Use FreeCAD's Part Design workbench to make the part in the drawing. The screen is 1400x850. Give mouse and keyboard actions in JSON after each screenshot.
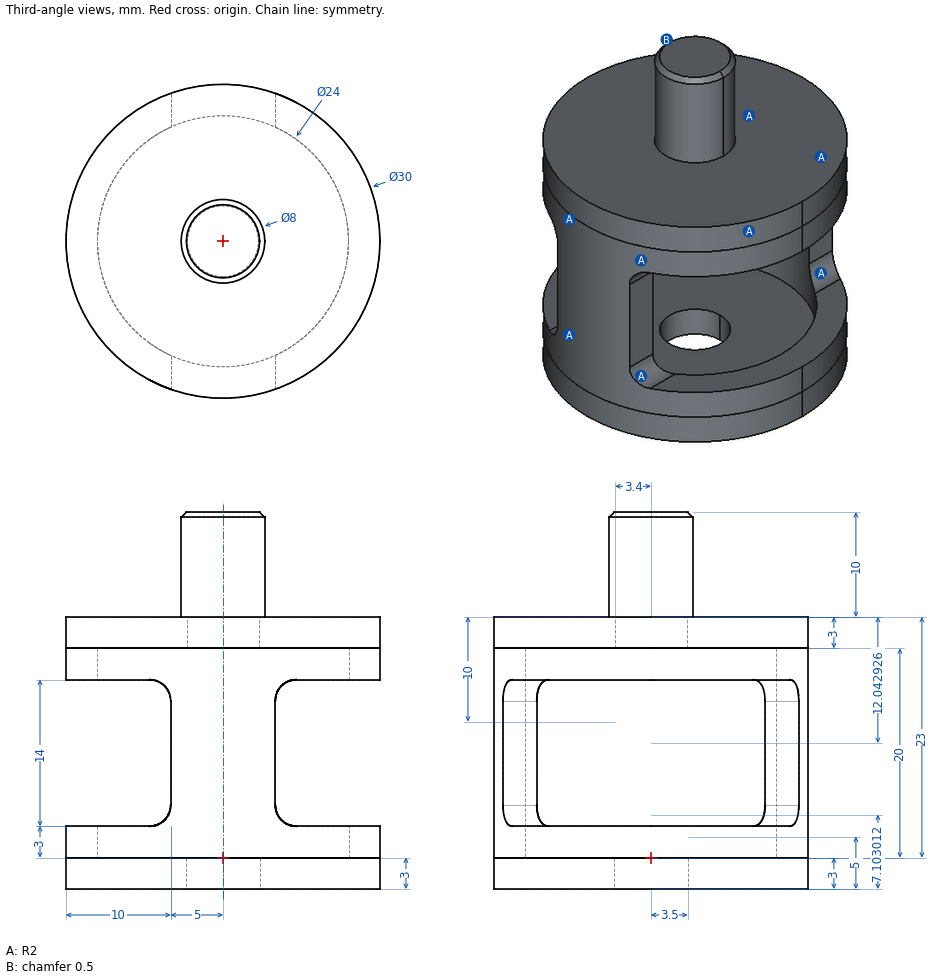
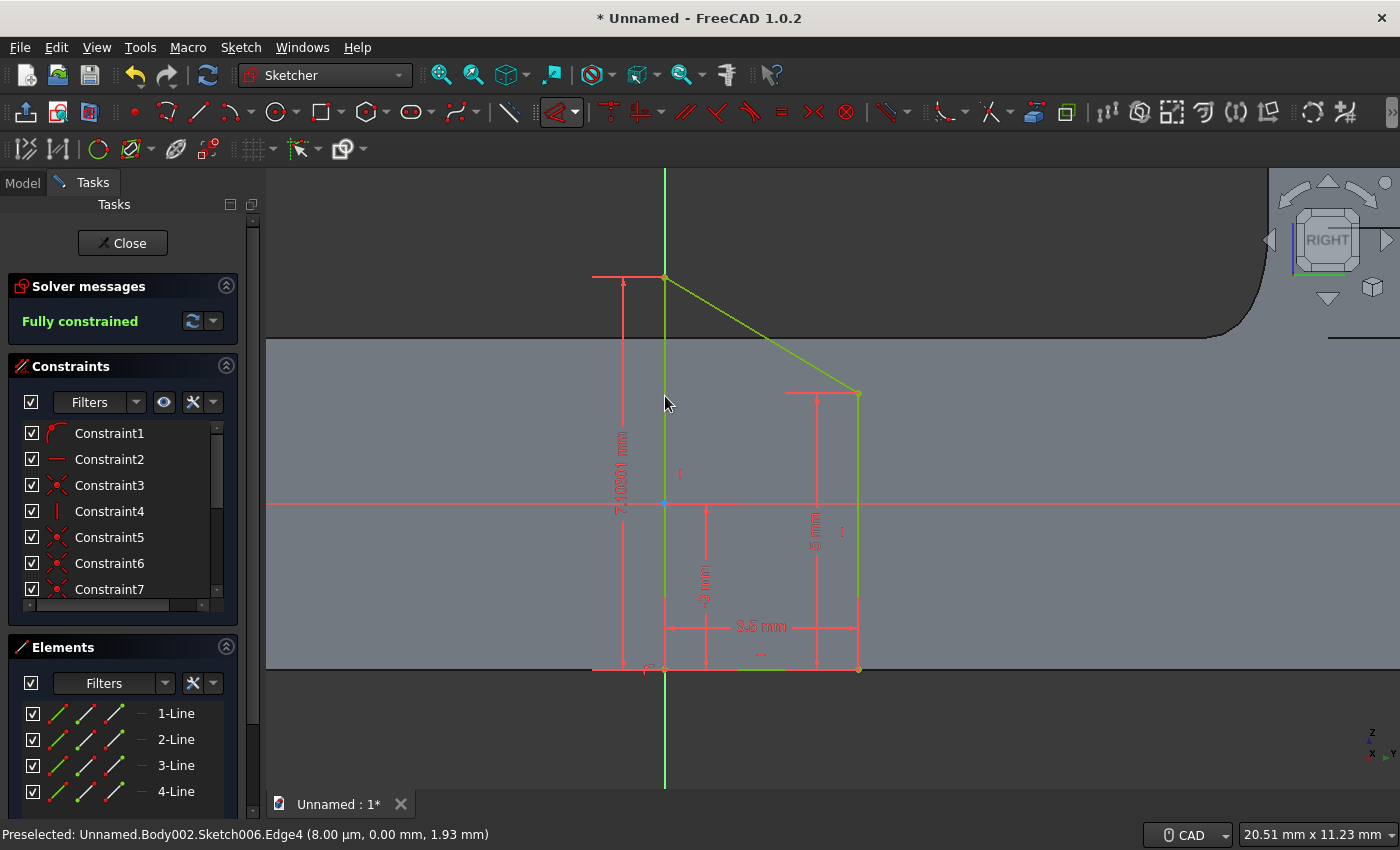
{"action": "left_click", "coordinate": [123, 243]}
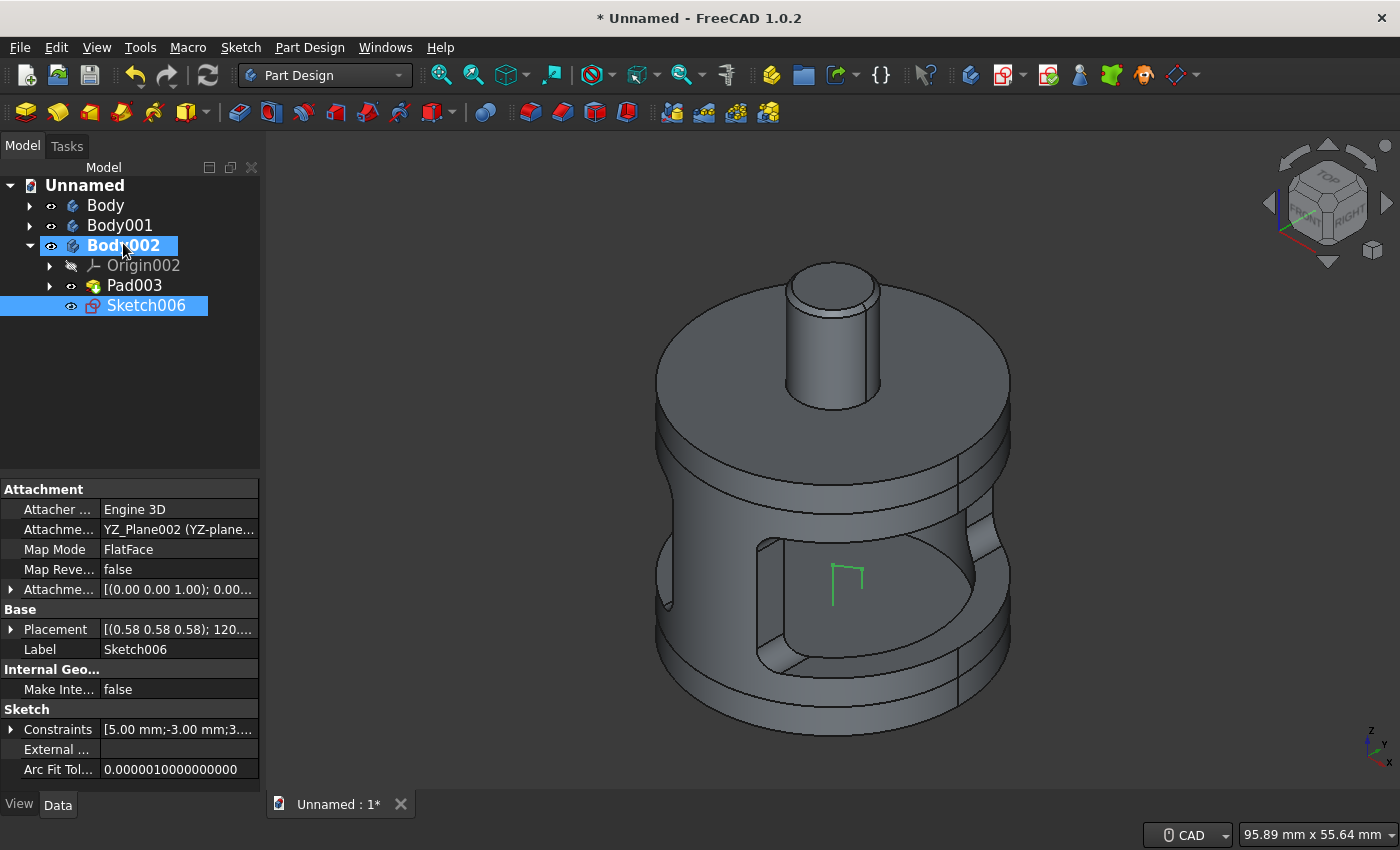
{"action": "left_click", "coordinate": [304, 112]}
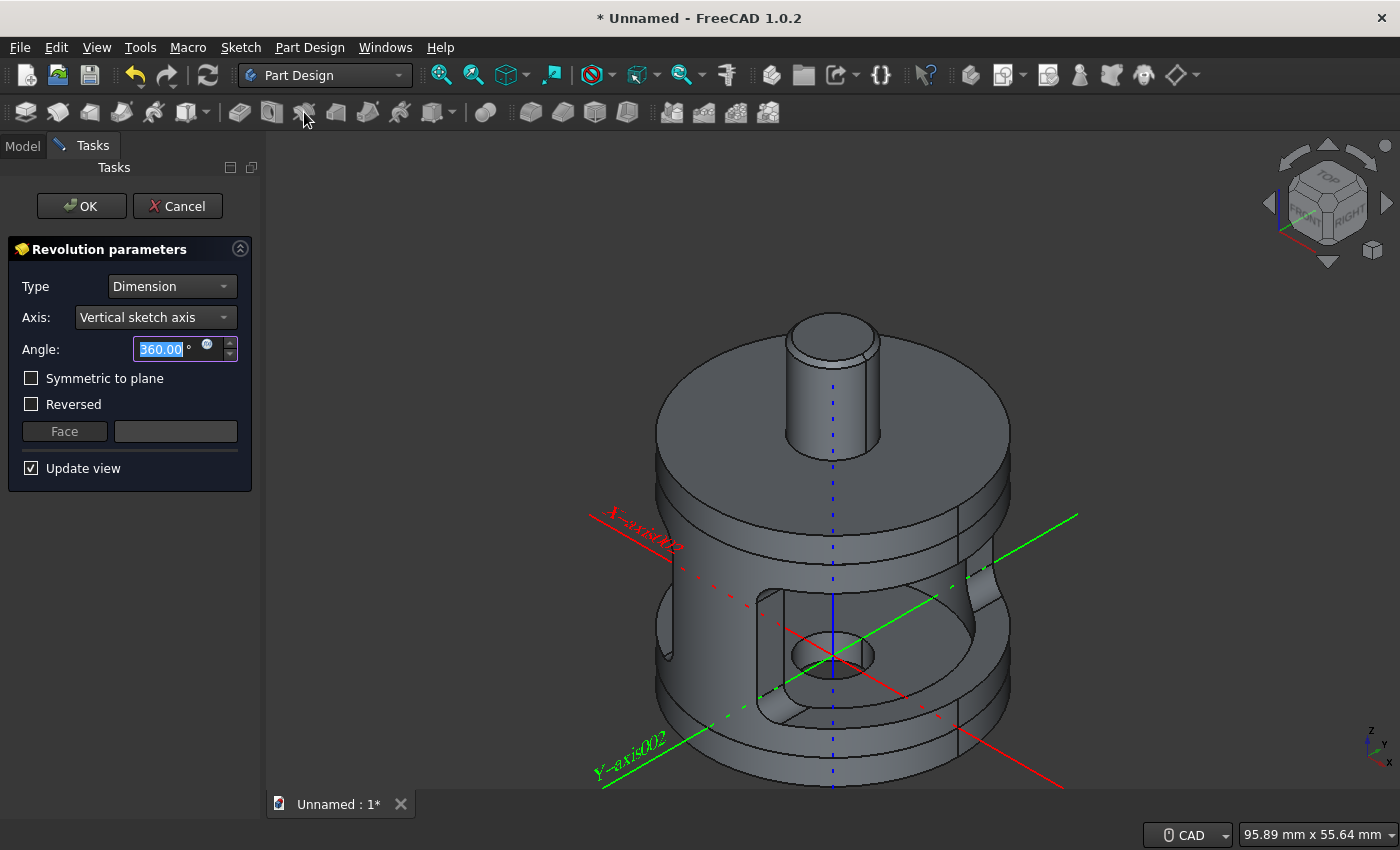
{"action": "left_click", "coordinate": [82, 206]}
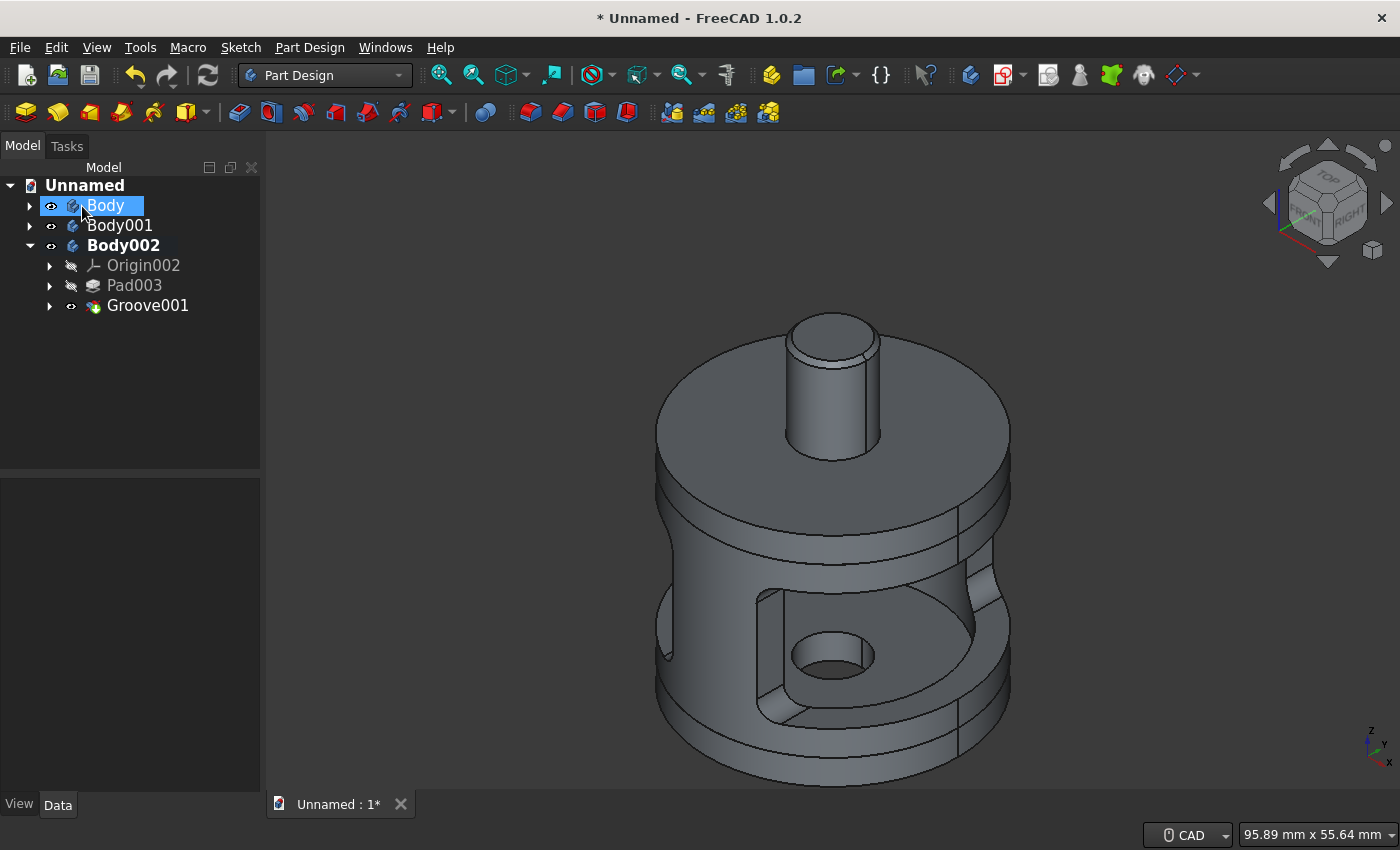
{"action": "left_click", "coordinate": [442, 76]}